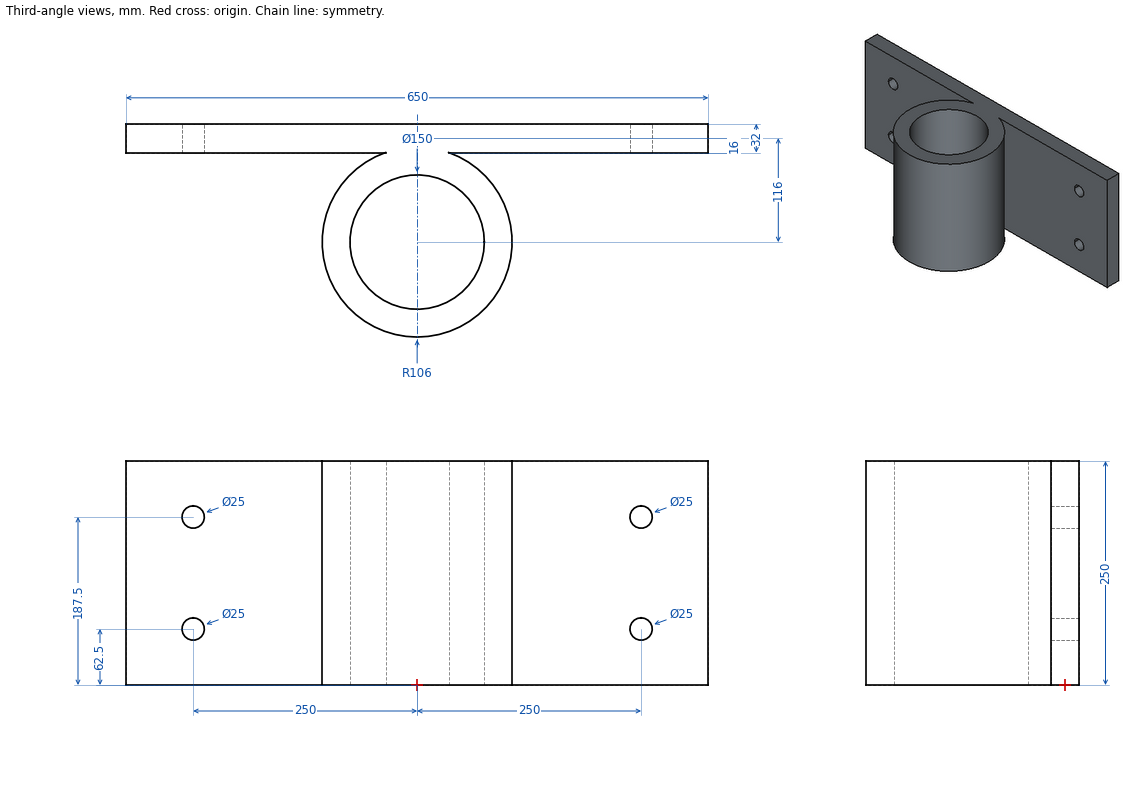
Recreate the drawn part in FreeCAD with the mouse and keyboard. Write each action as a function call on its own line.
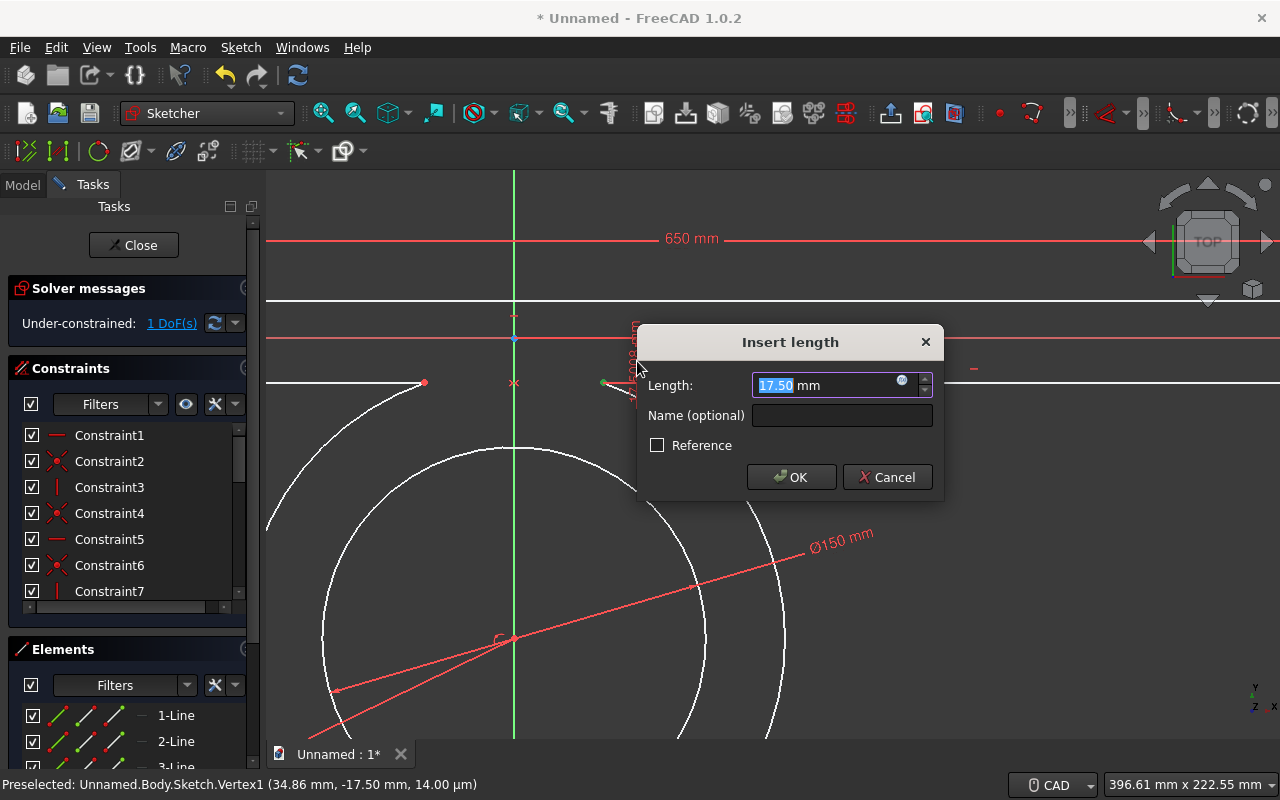
text(16)
key(Return)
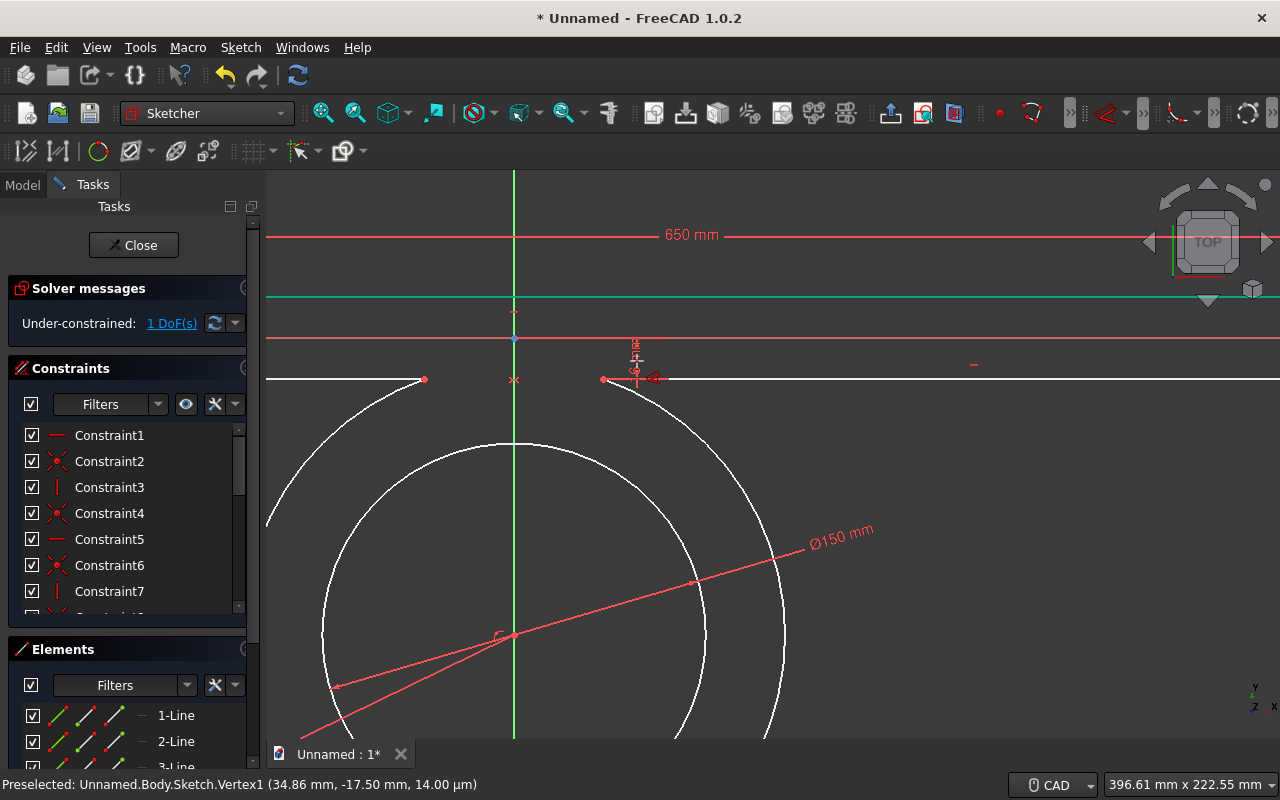
click(514, 635)
click(548, 487)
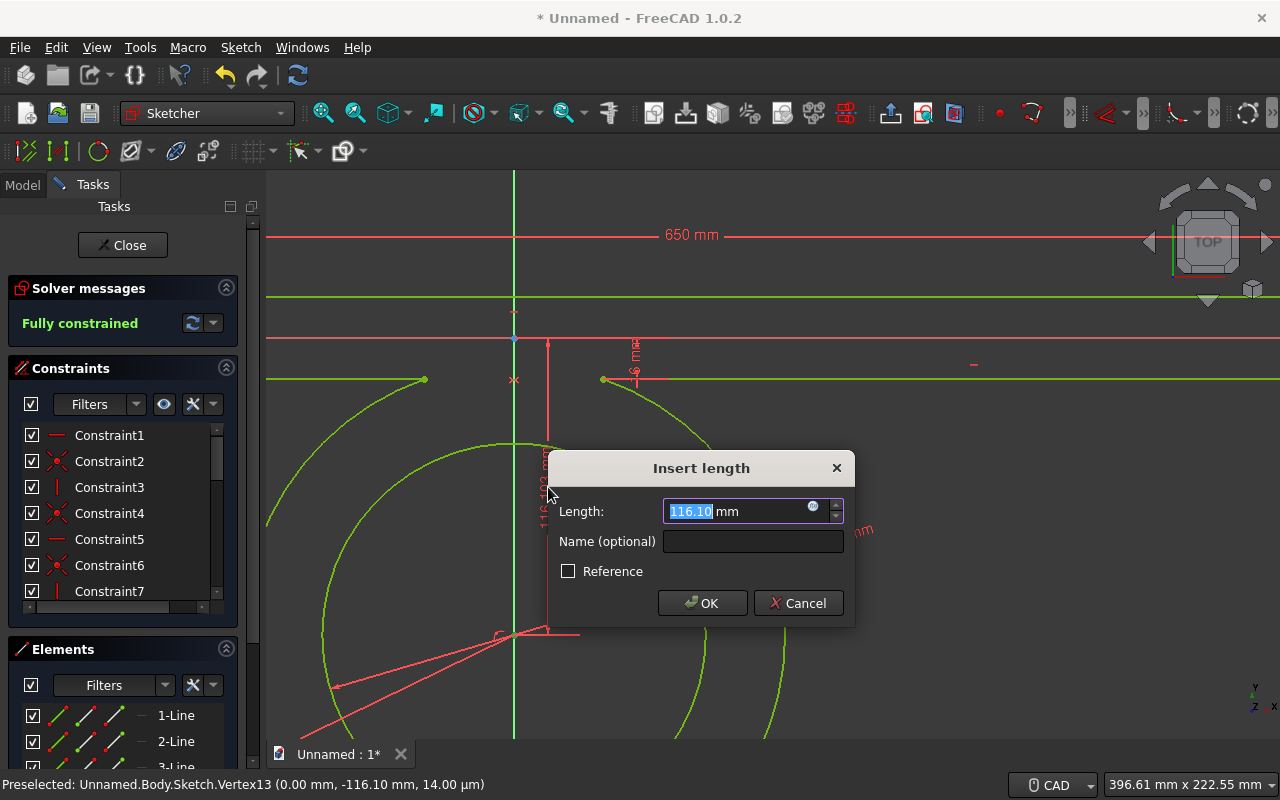
text(116)
key(Return)
key(Escape)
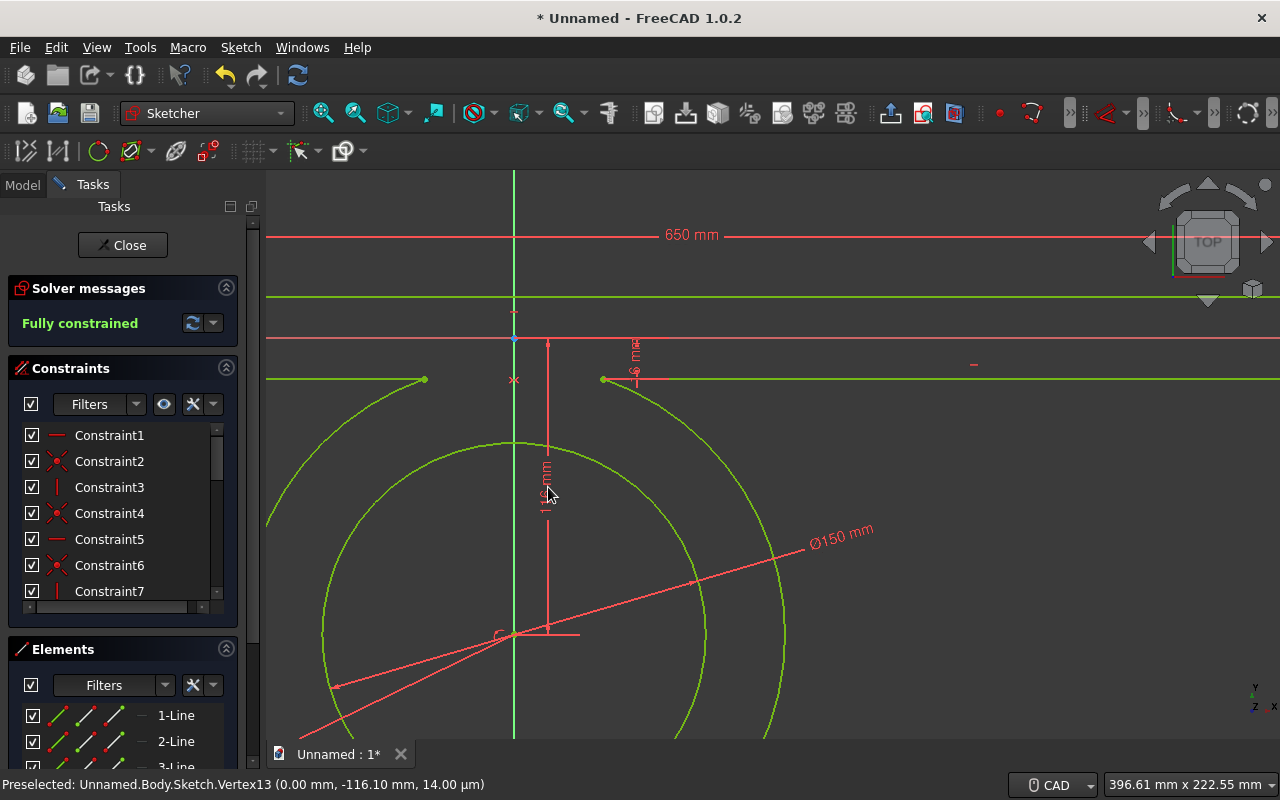
click(123, 245)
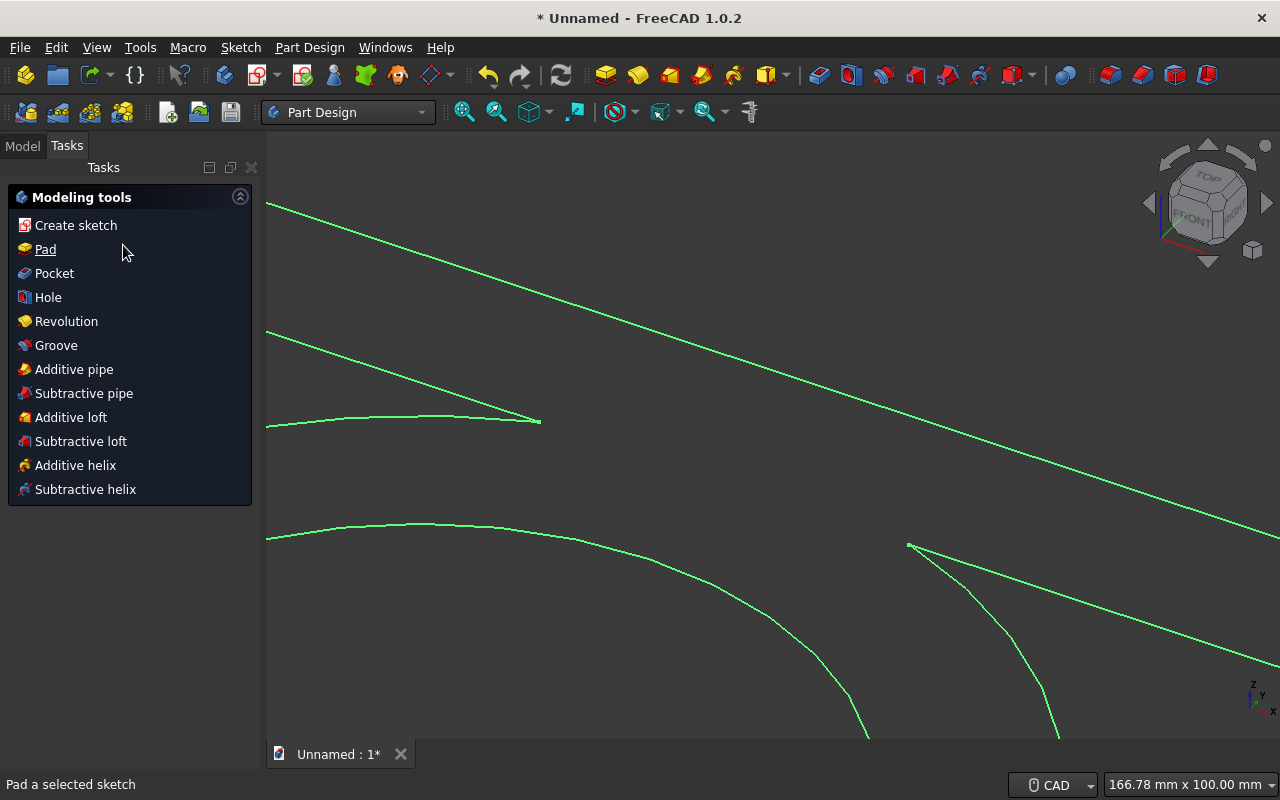
click(606, 76)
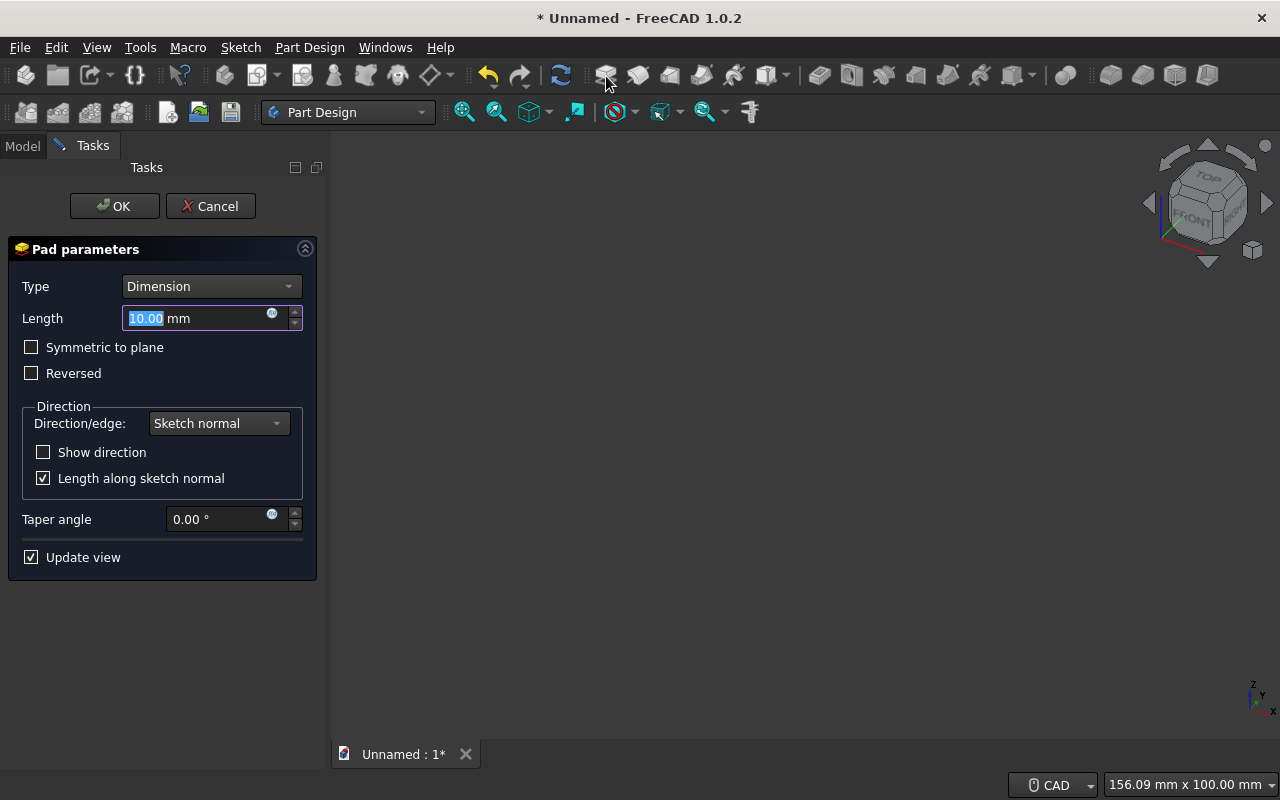
text(250)
key(Tab)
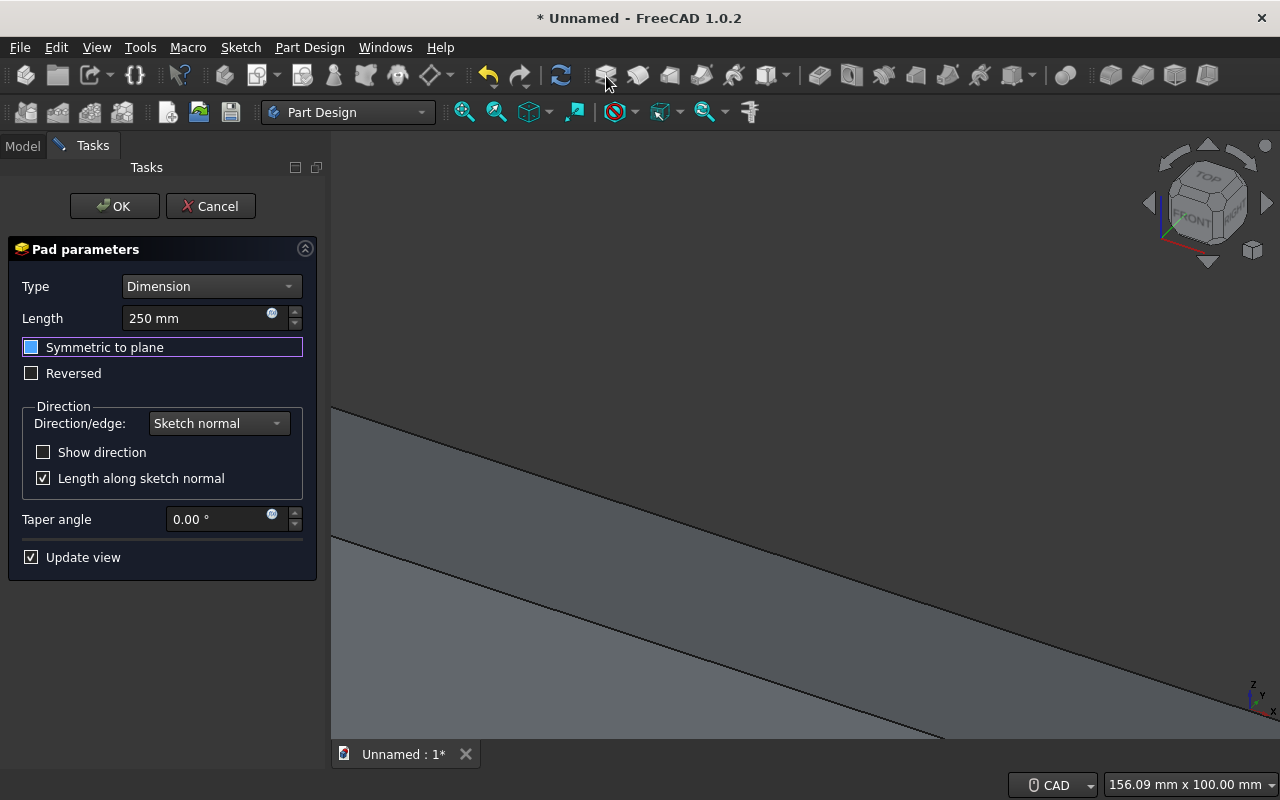
click(115, 206)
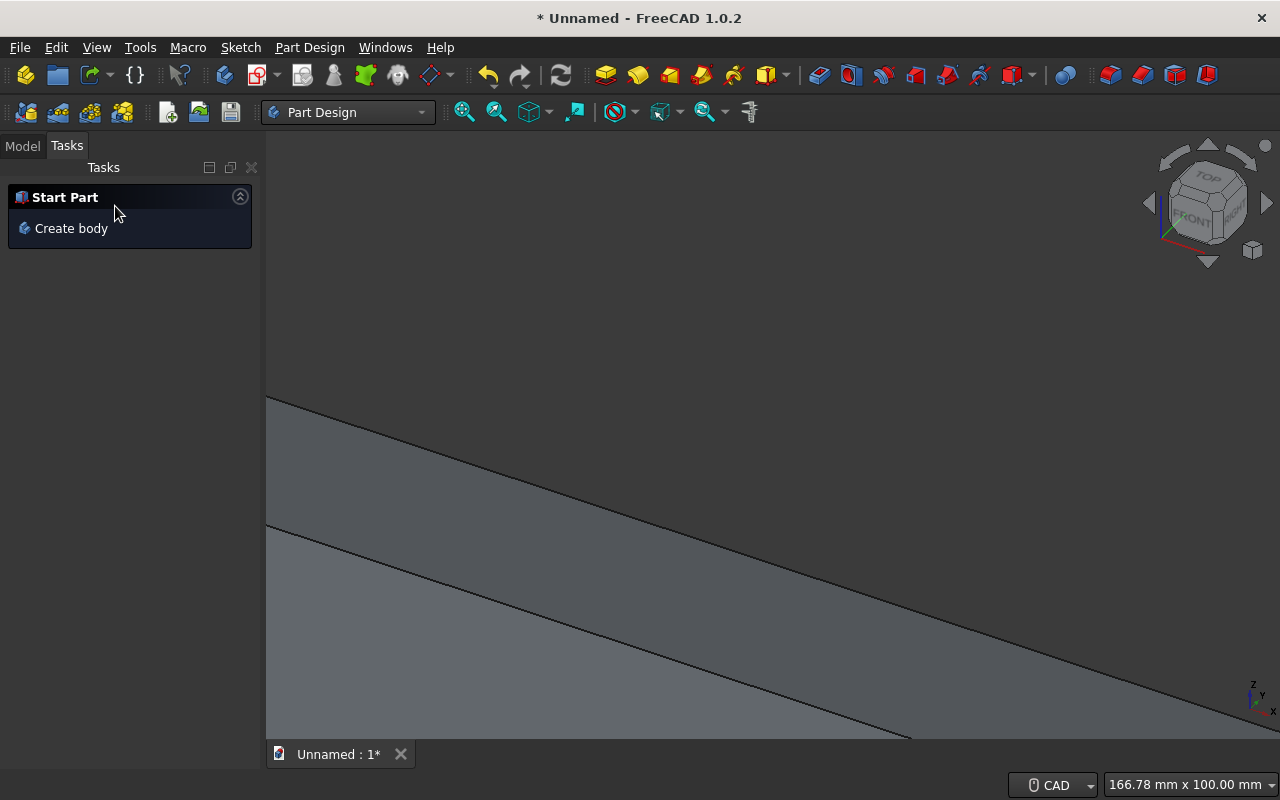
key(v)
key(f)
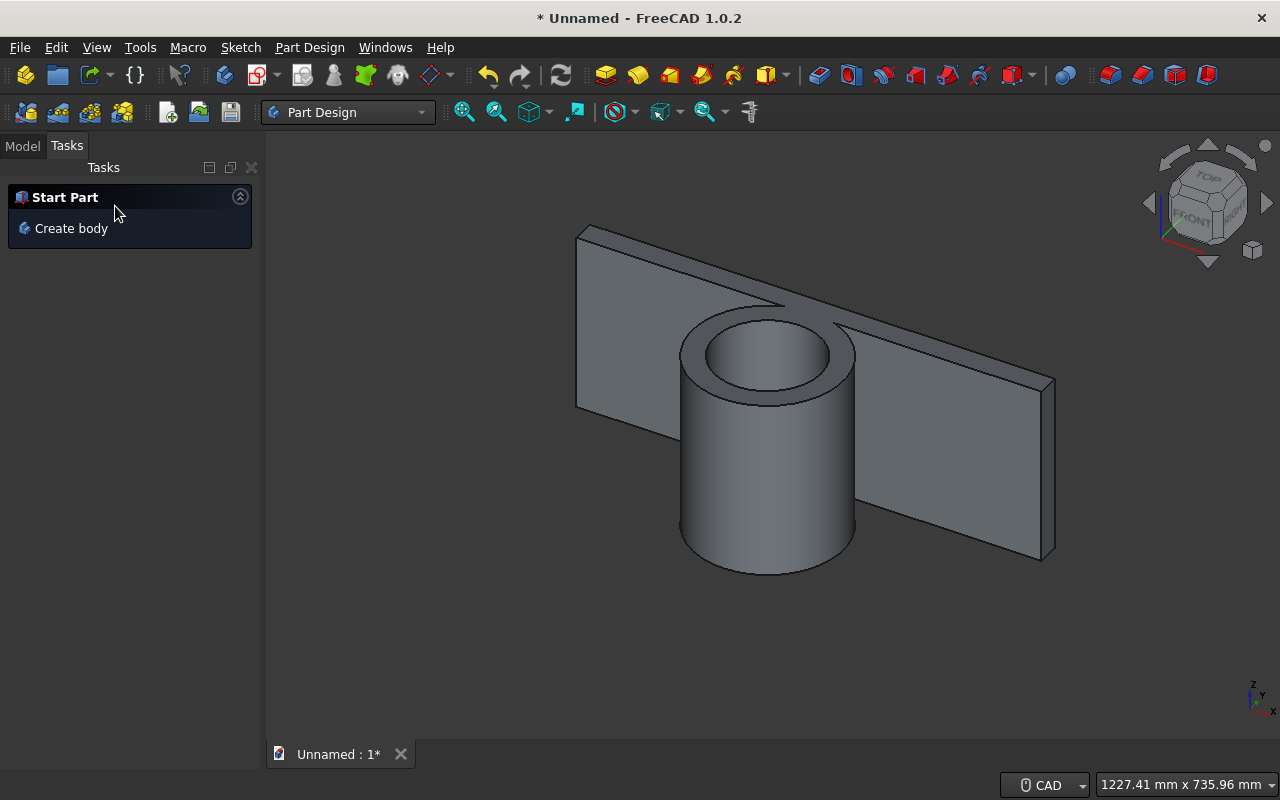
key(4)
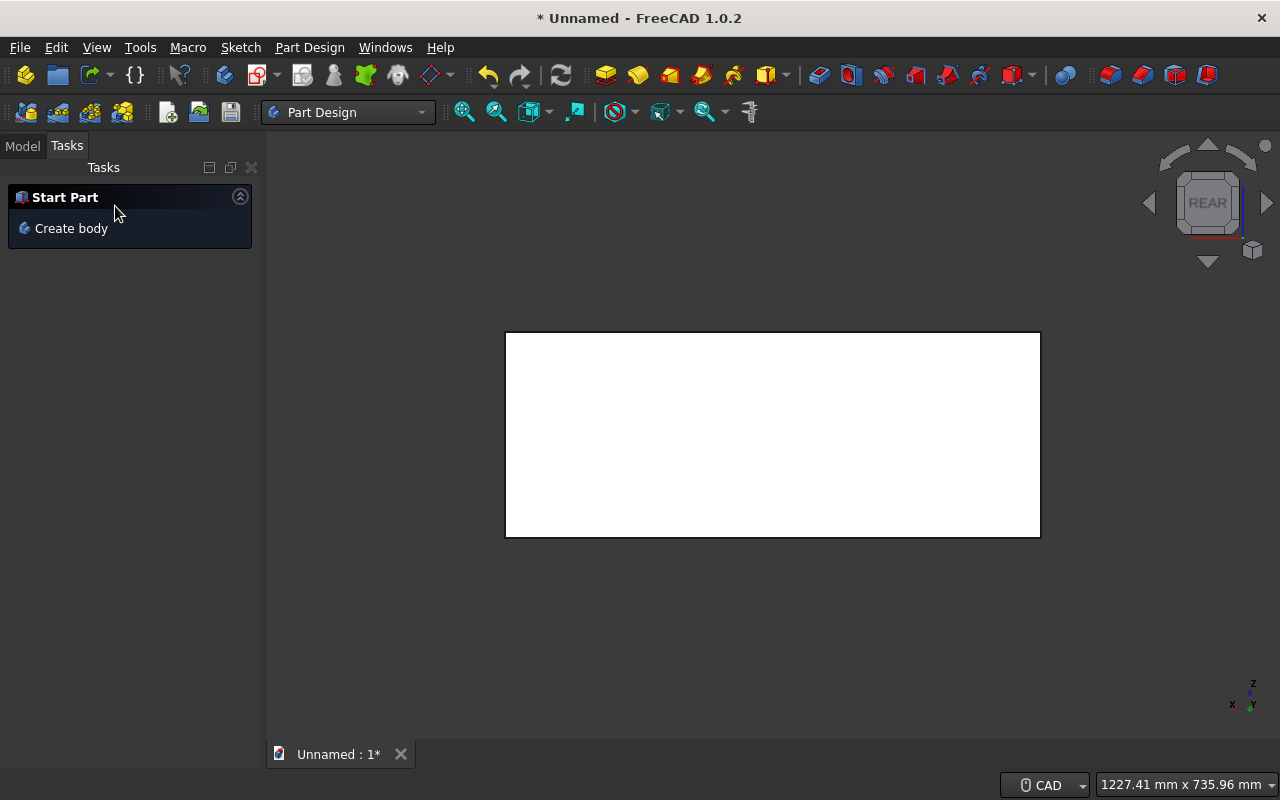
click(620, 434)